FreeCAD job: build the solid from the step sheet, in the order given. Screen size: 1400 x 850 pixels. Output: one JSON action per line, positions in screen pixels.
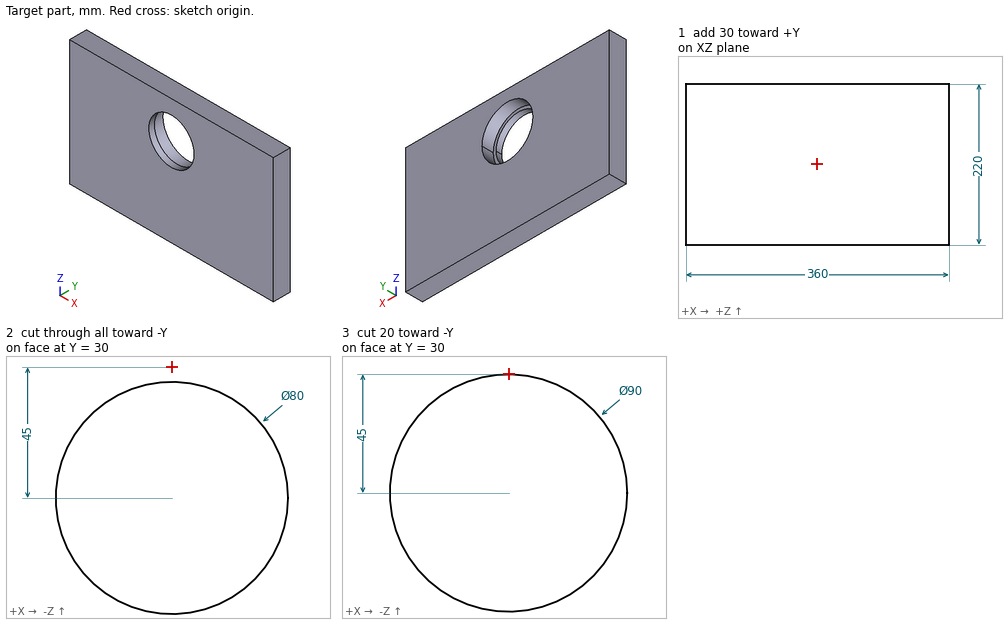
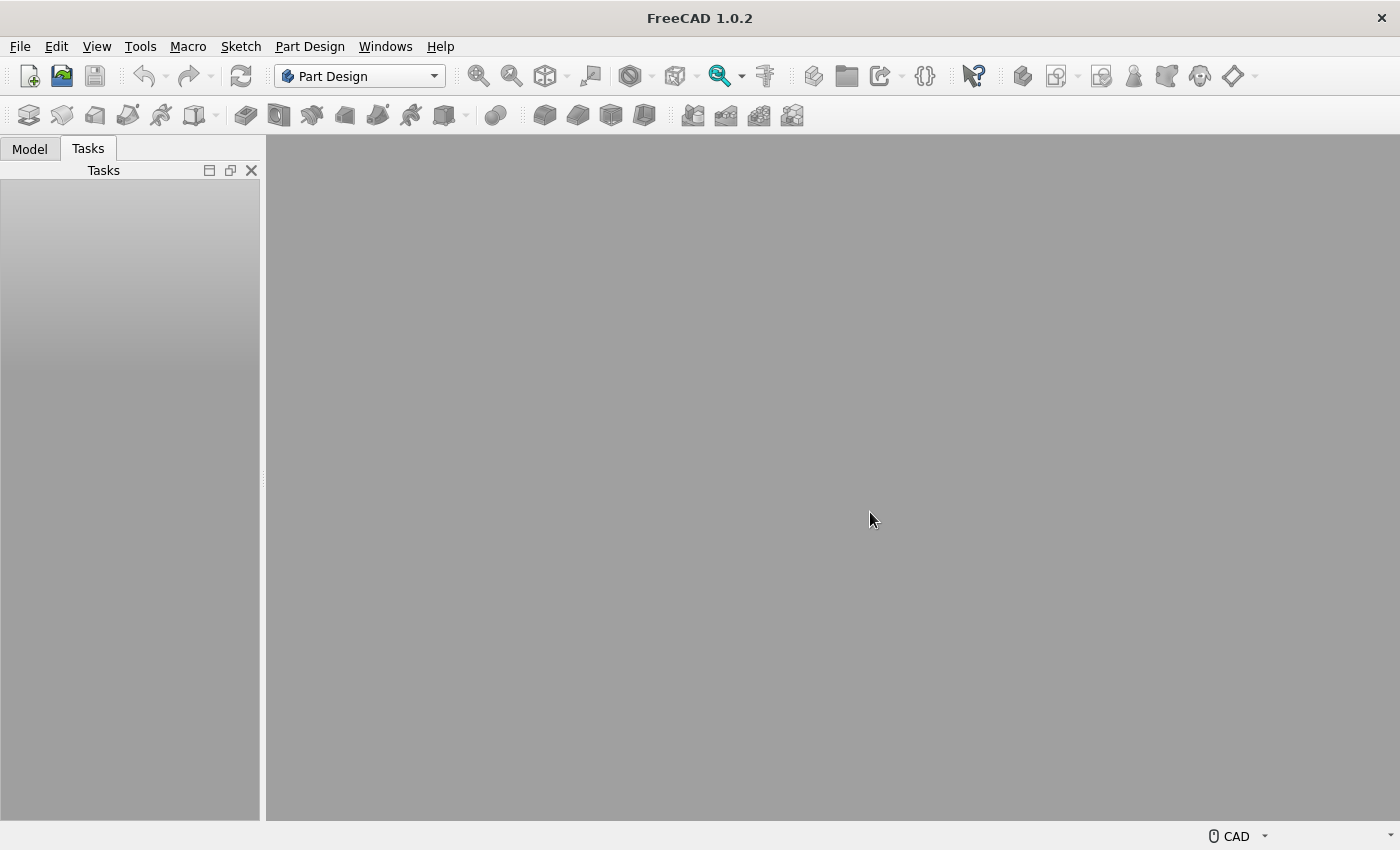
{"action": "left_click", "coordinate": [29, 76]}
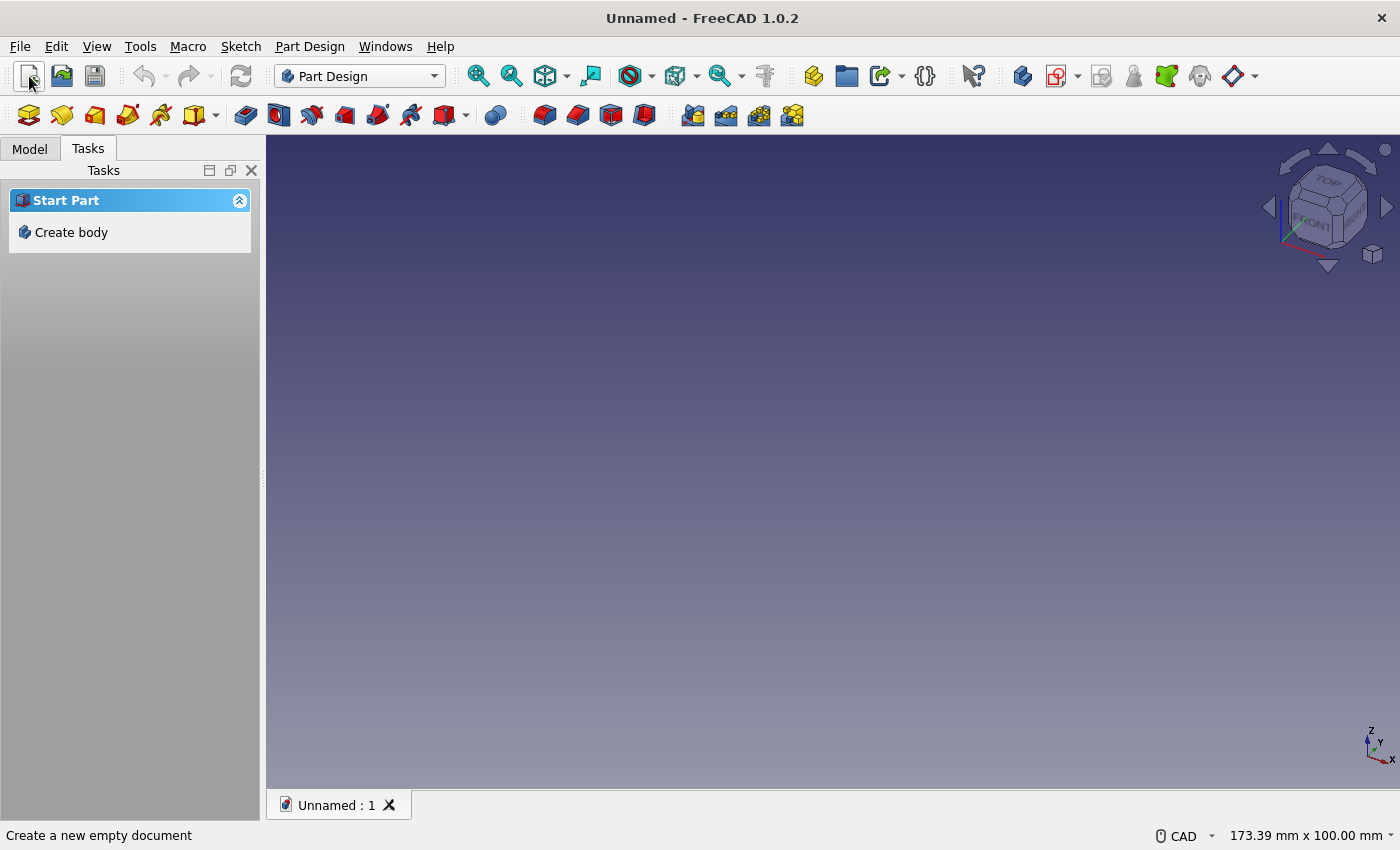
{"action": "left_click", "coordinate": [1056, 76]}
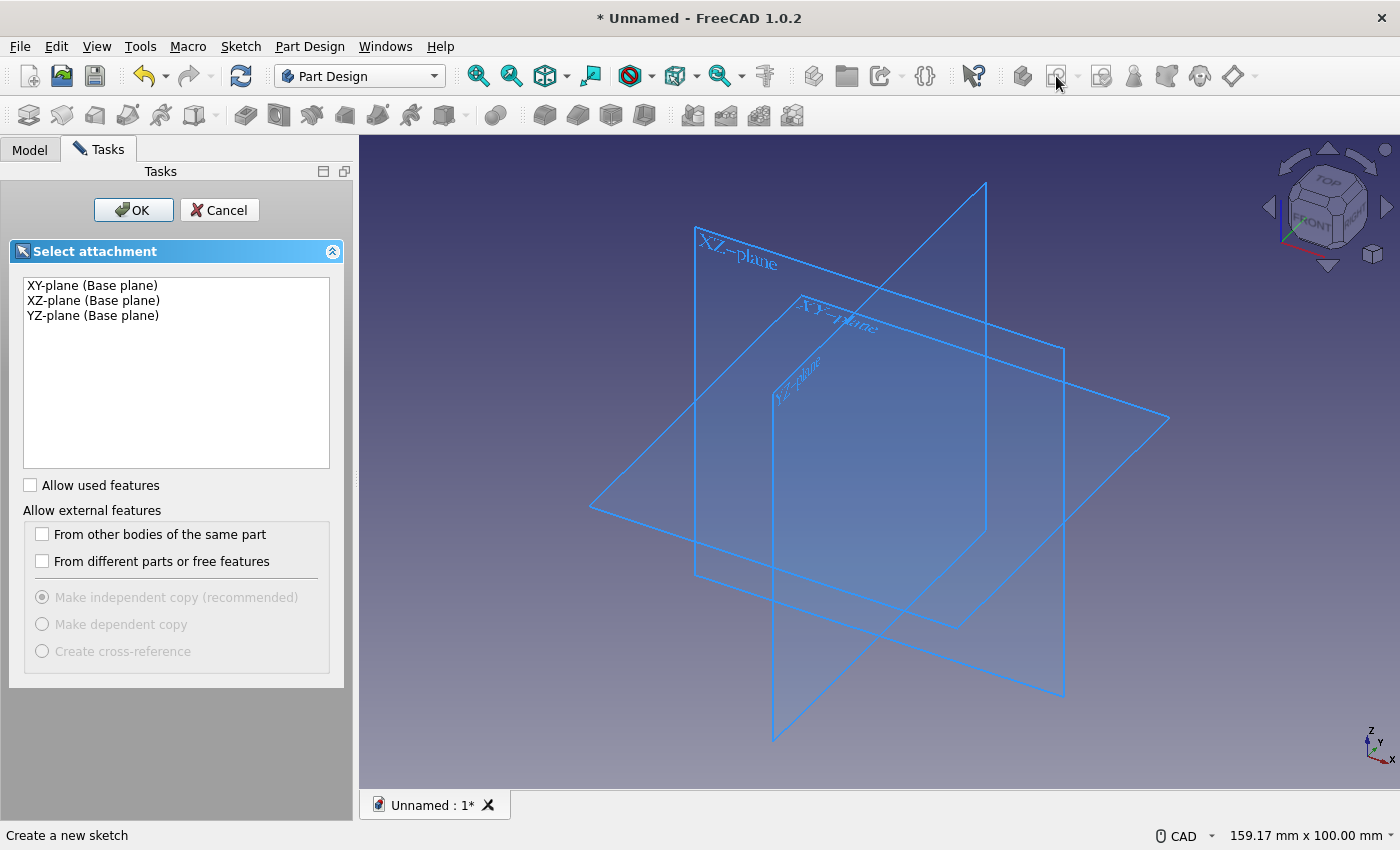
{"action": "left_click", "coordinate": [84, 300]}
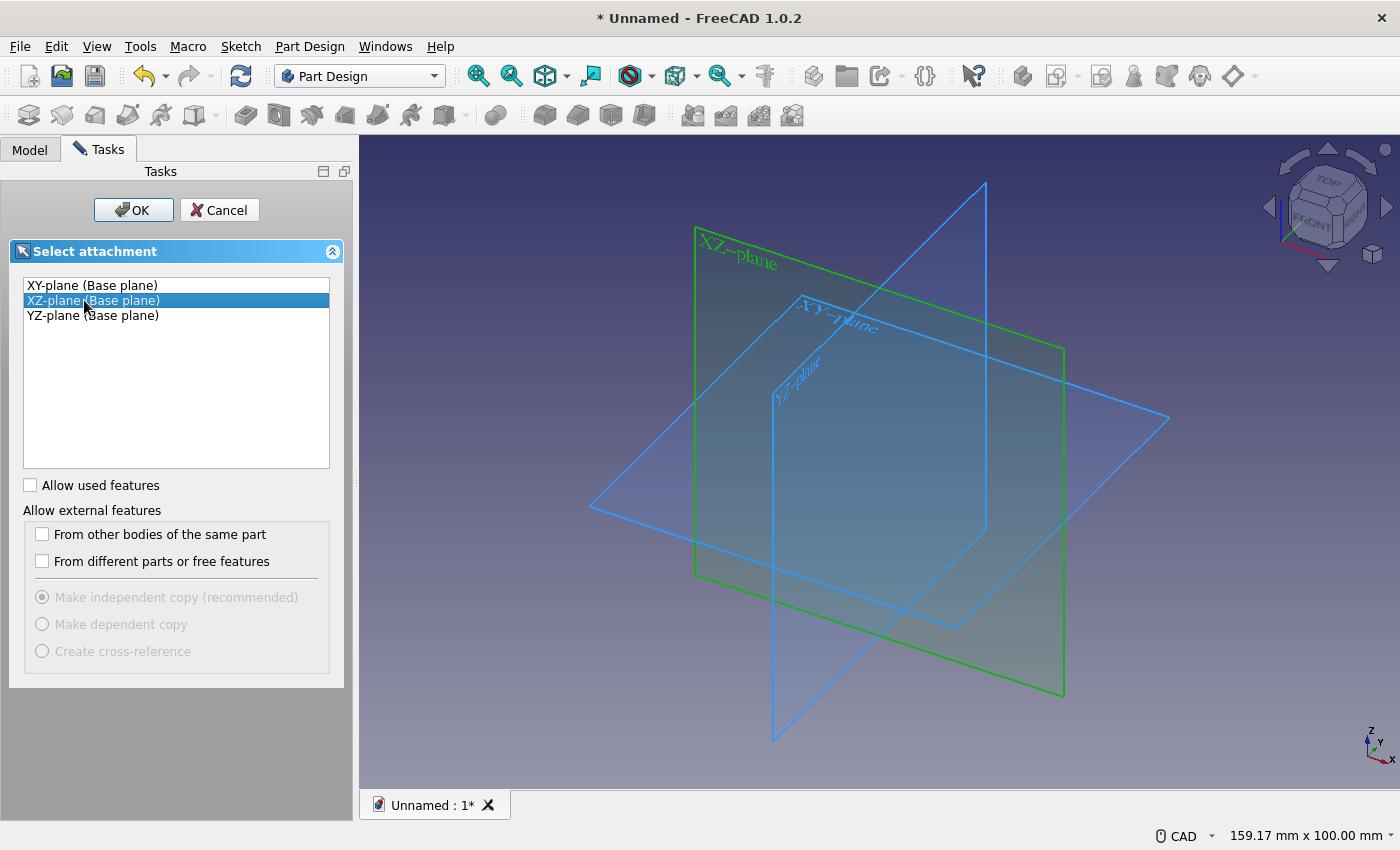
{"action": "left_click", "coordinate": [134, 210]}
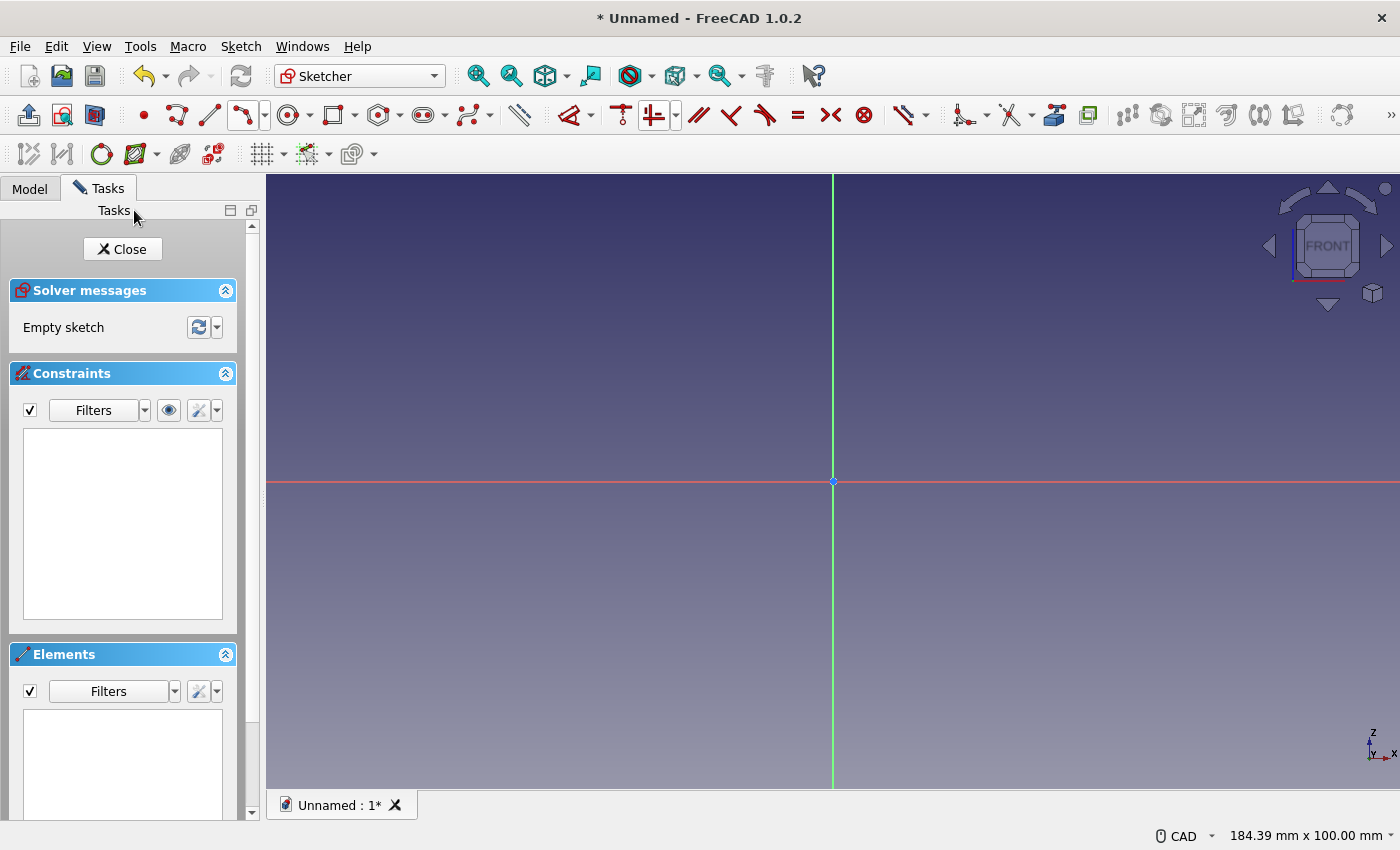
{"action": "scroll", "coordinate": [735, 481], "scroll_direction": "down", "scroll_amount": 6}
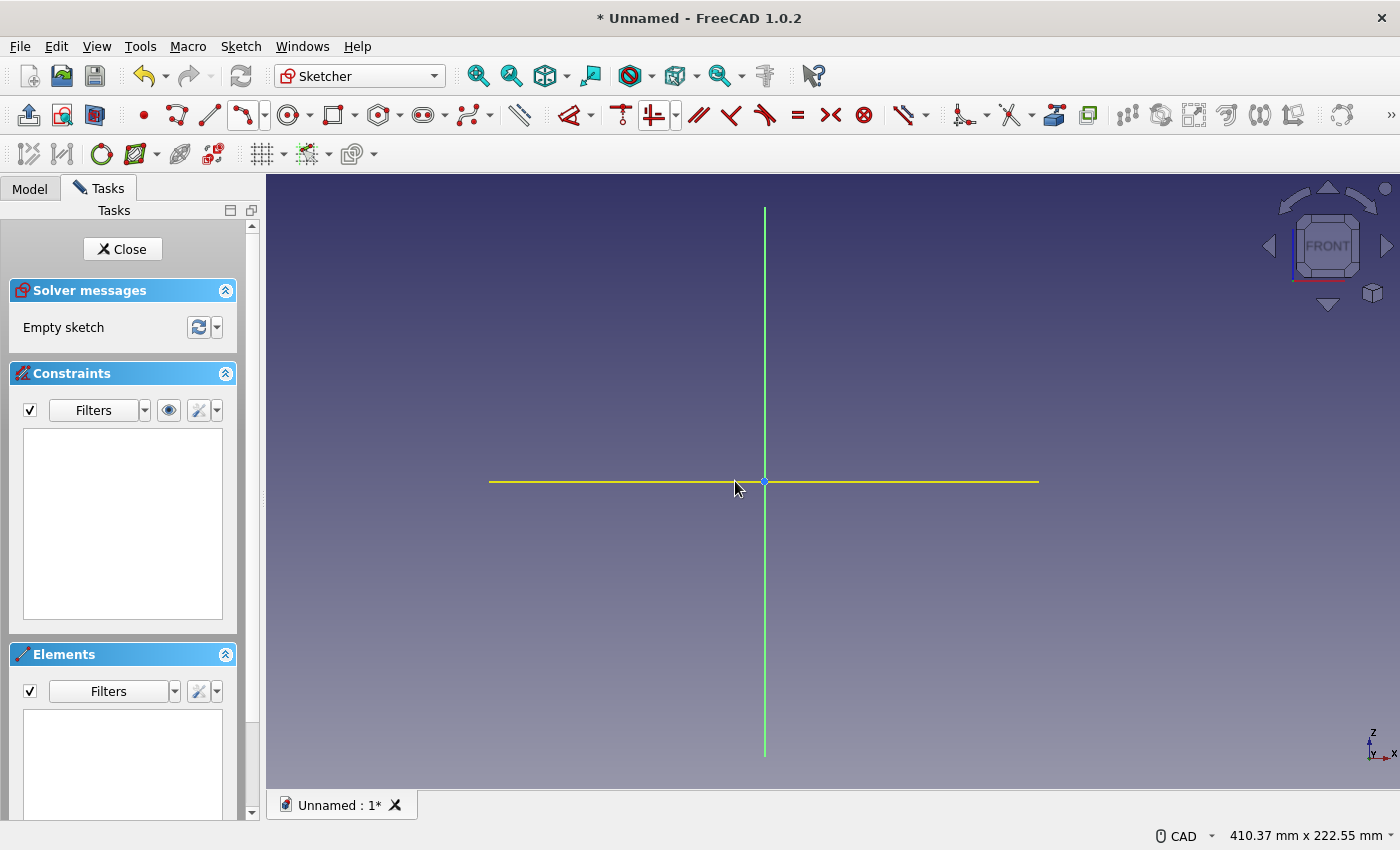
{"action": "key", "text": "g v"}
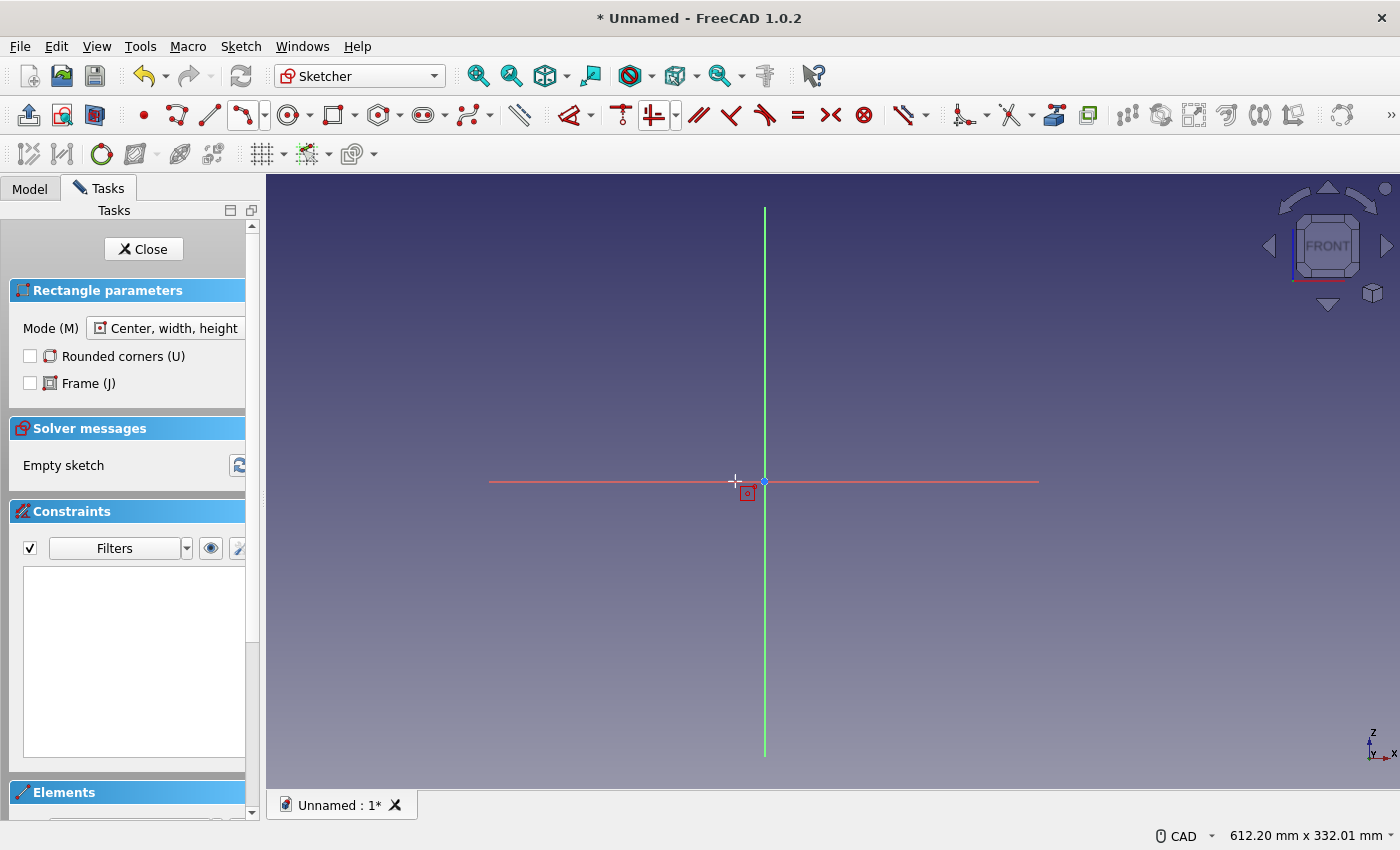
{"action": "left_click", "coordinate": [765, 482]}
{"action": "mouse_move", "coordinate": [1098, 278]}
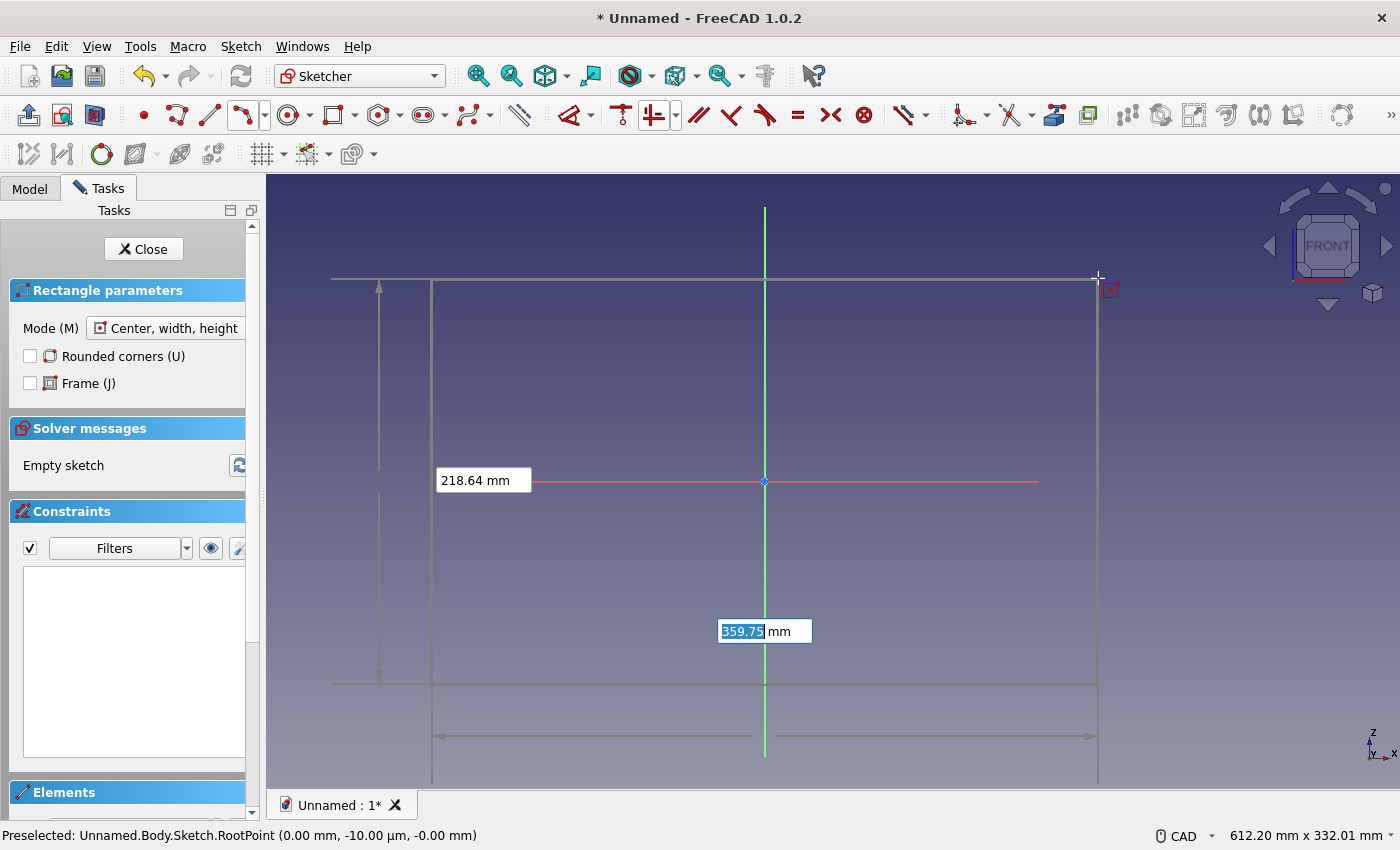
{"action": "type", "text": "360"}
{"action": "key", "text": "Tab"}
{"action": "type", "text": "220"}
{"action": "key", "text": "Return"}
{"action": "key", "text": "Escape"}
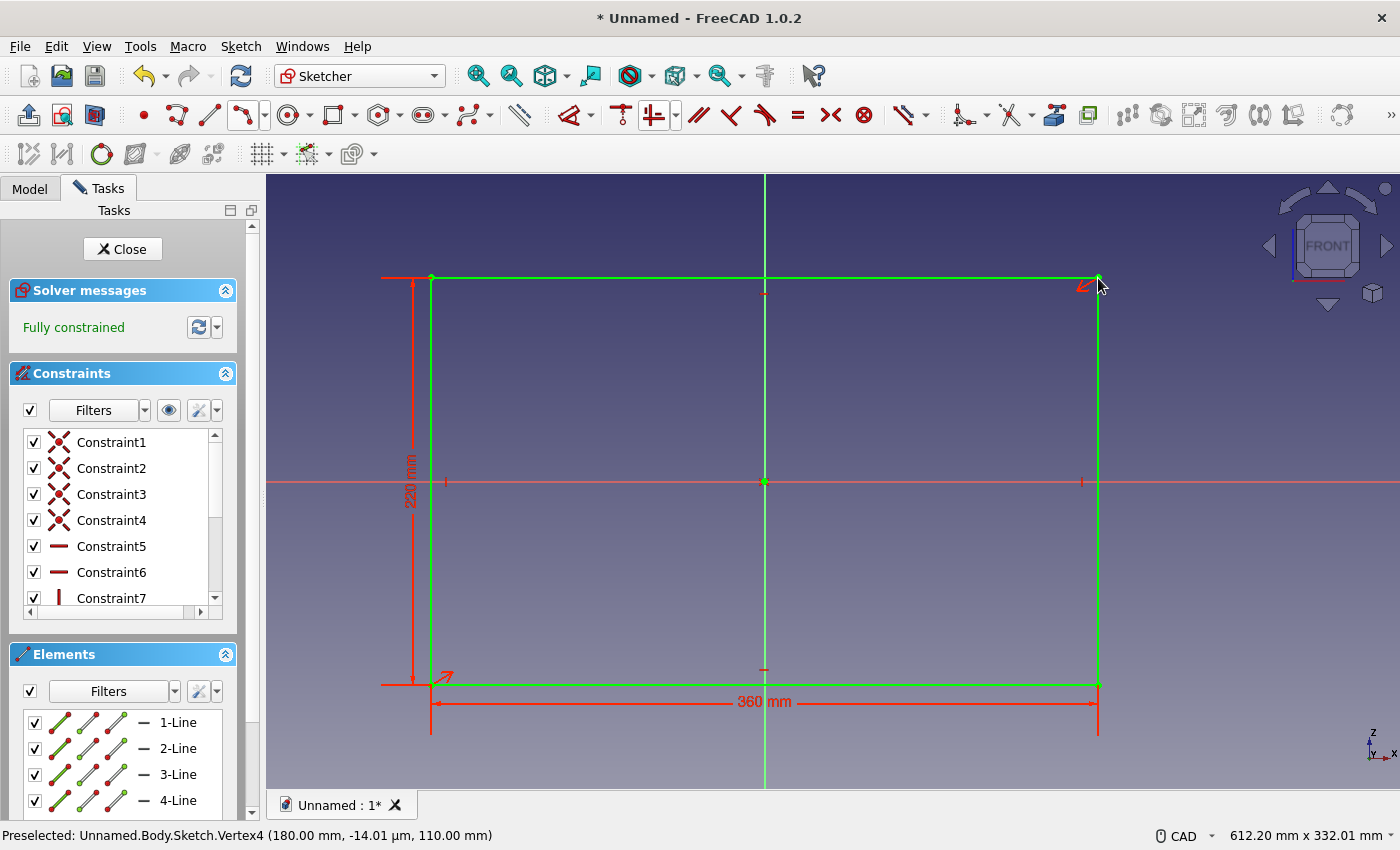
{"action": "left_click", "coordinate": [123, 249]}